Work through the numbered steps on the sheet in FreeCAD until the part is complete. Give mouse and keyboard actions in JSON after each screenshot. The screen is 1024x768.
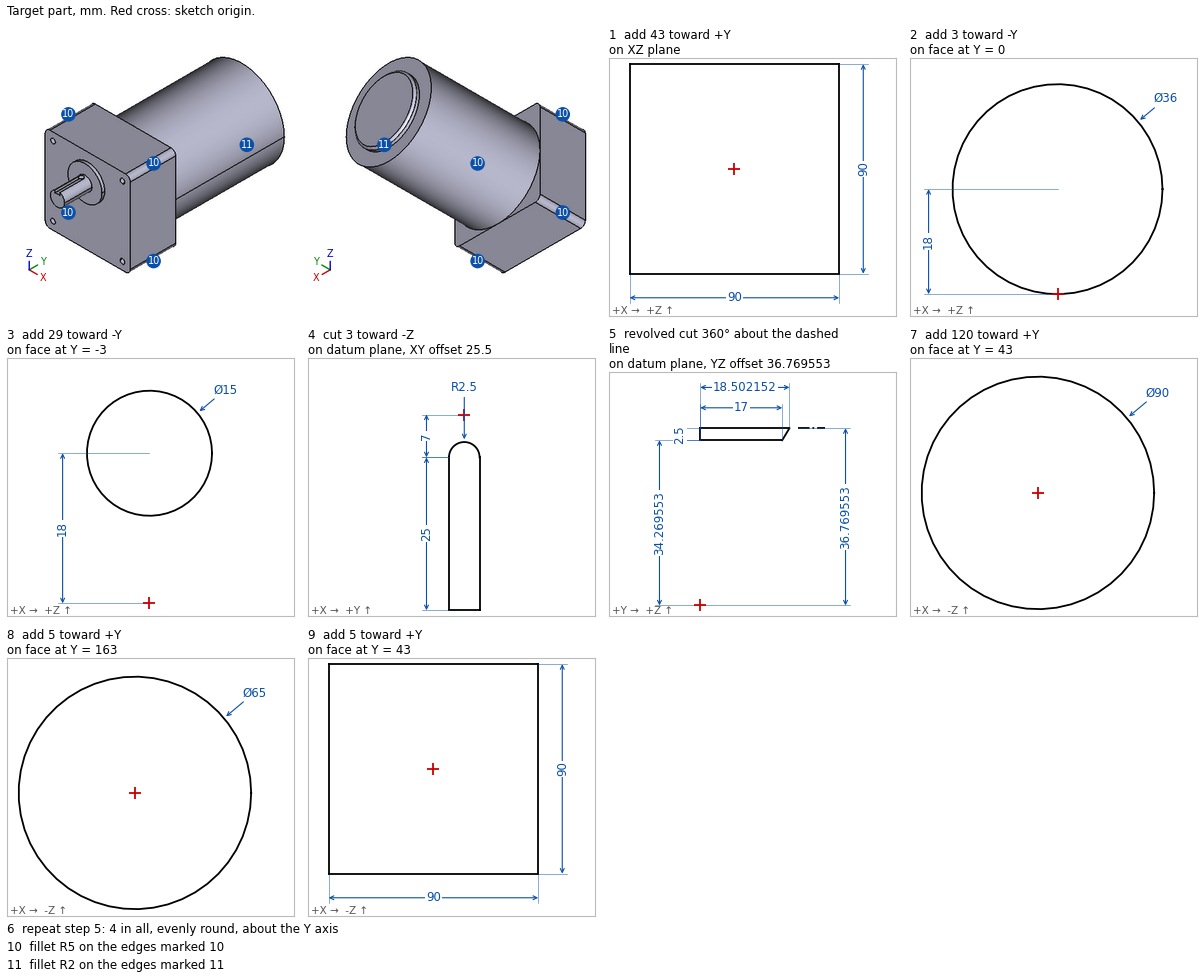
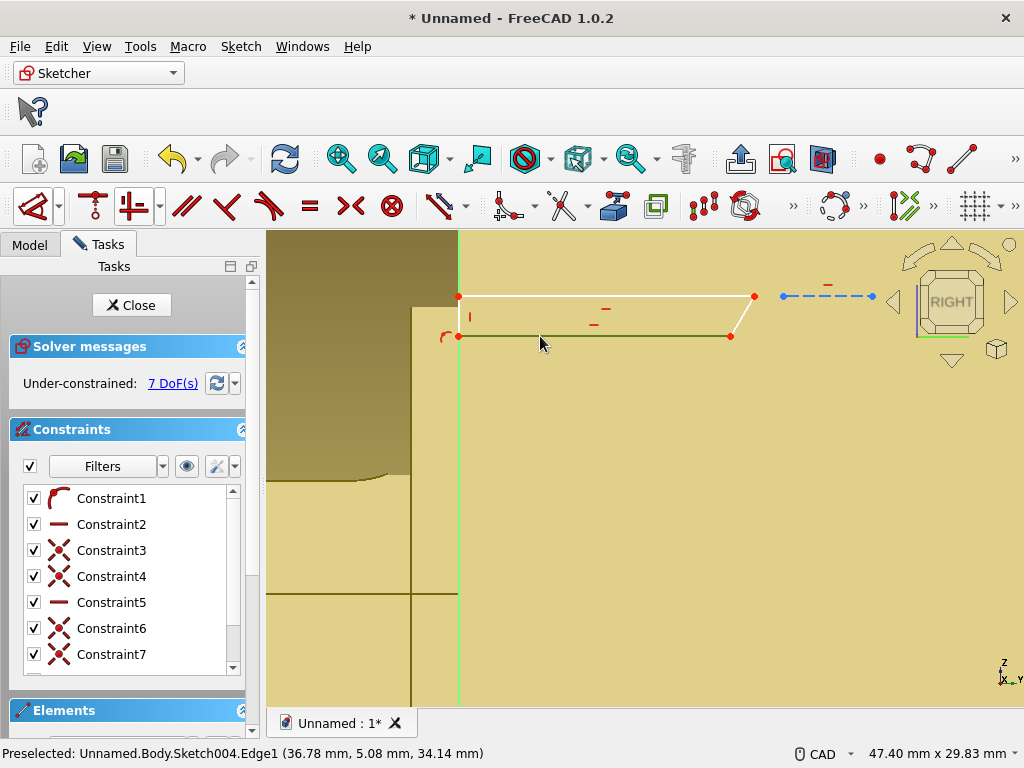
{"action": "left_click", "coordinate": [58, 206]}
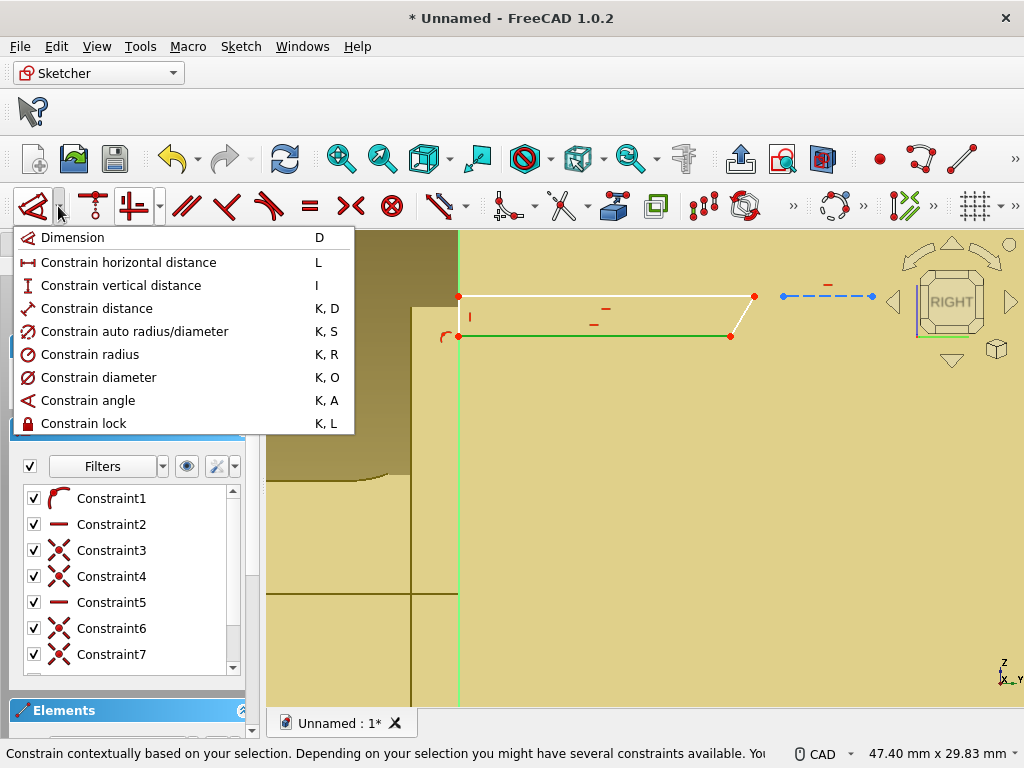
{"action": "left_click", "coordinate": [184, 262]}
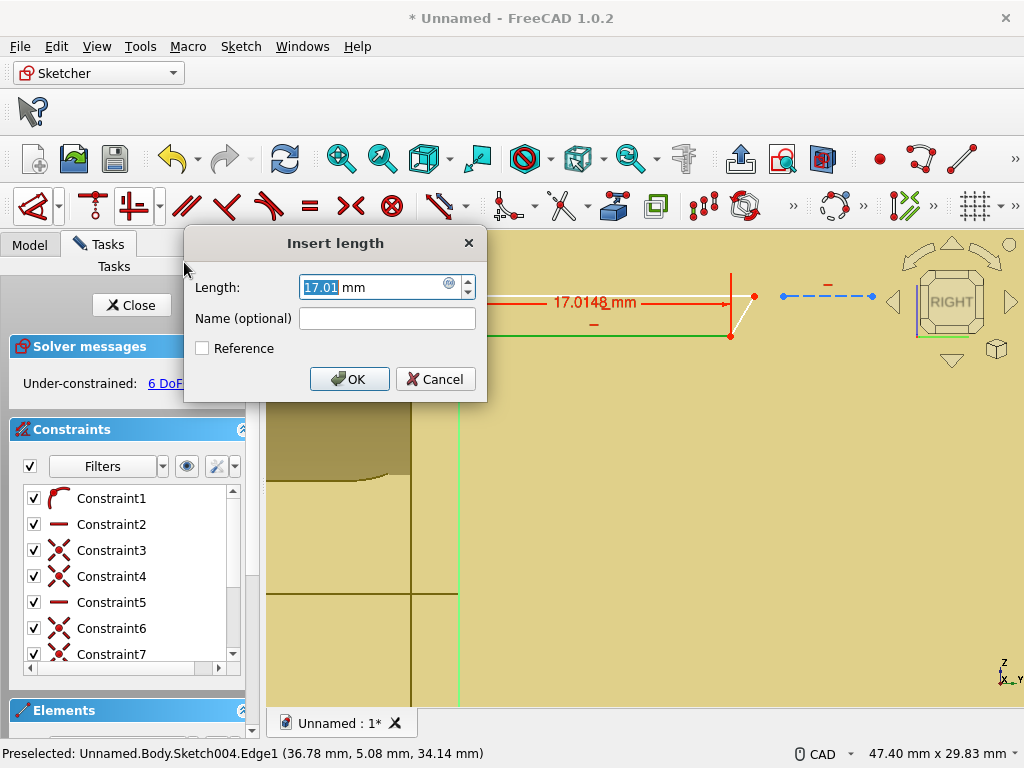
{"action": "type", "text": "17"}
{"action": "key", "text": "Return"}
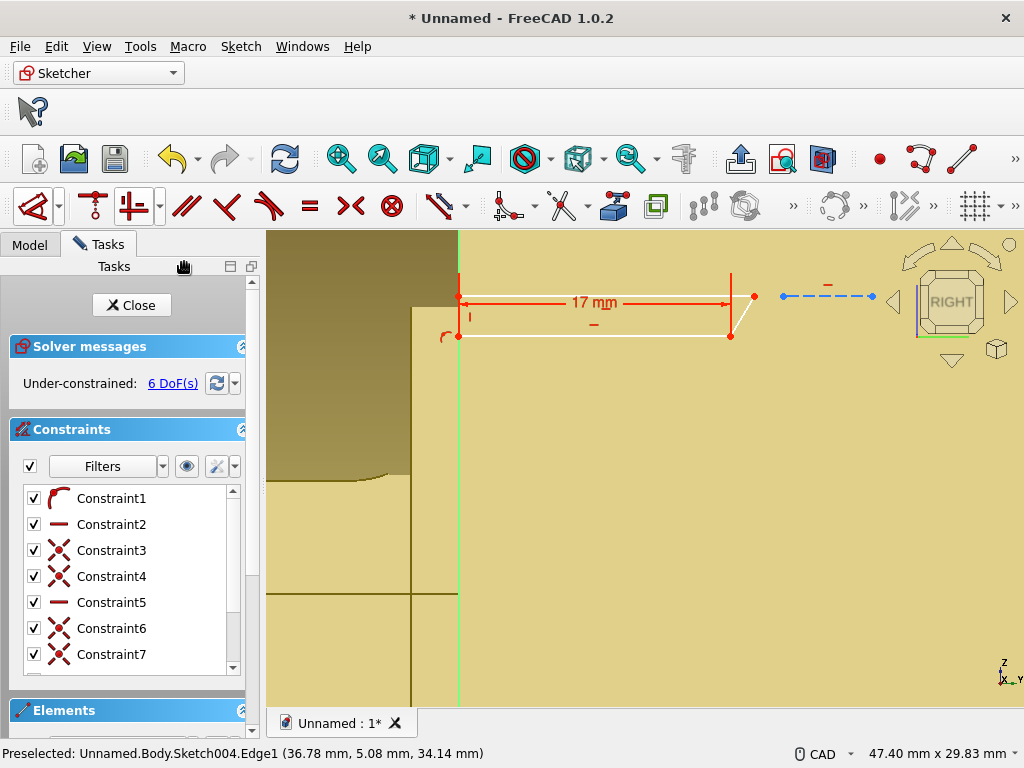
{"action": "left_click", "coordinate": [459, 308]}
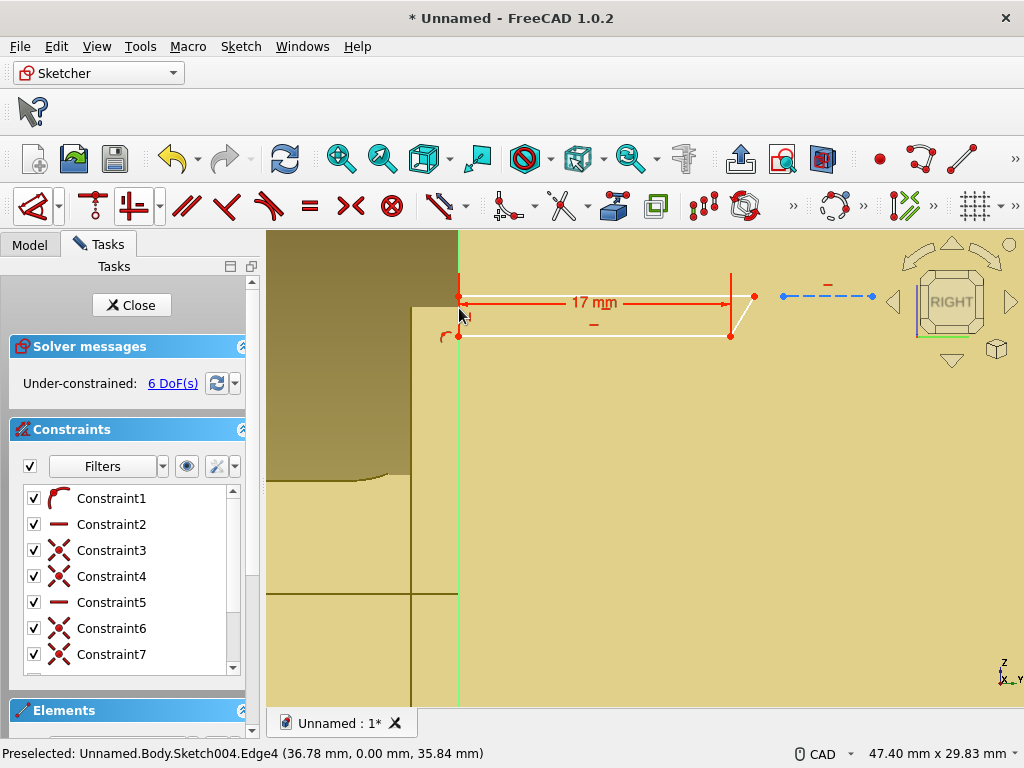
{"action": "key", "text": "i"}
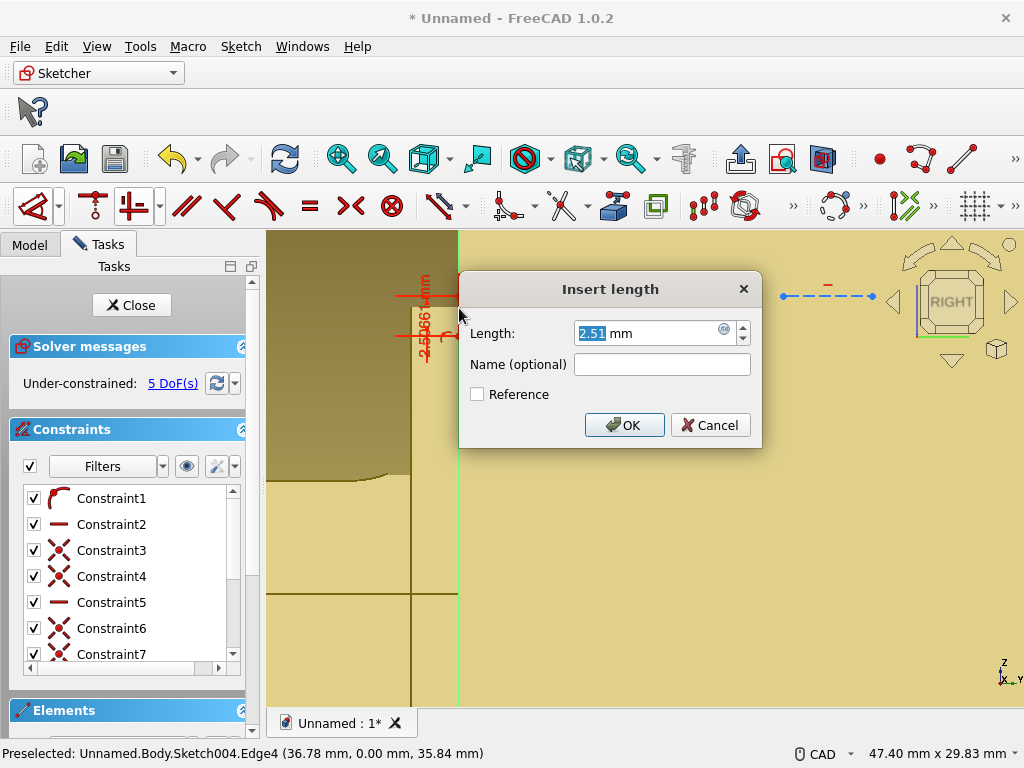
{"action": "type", "text": "2.5"}
{"action": "key", "text": "Return"}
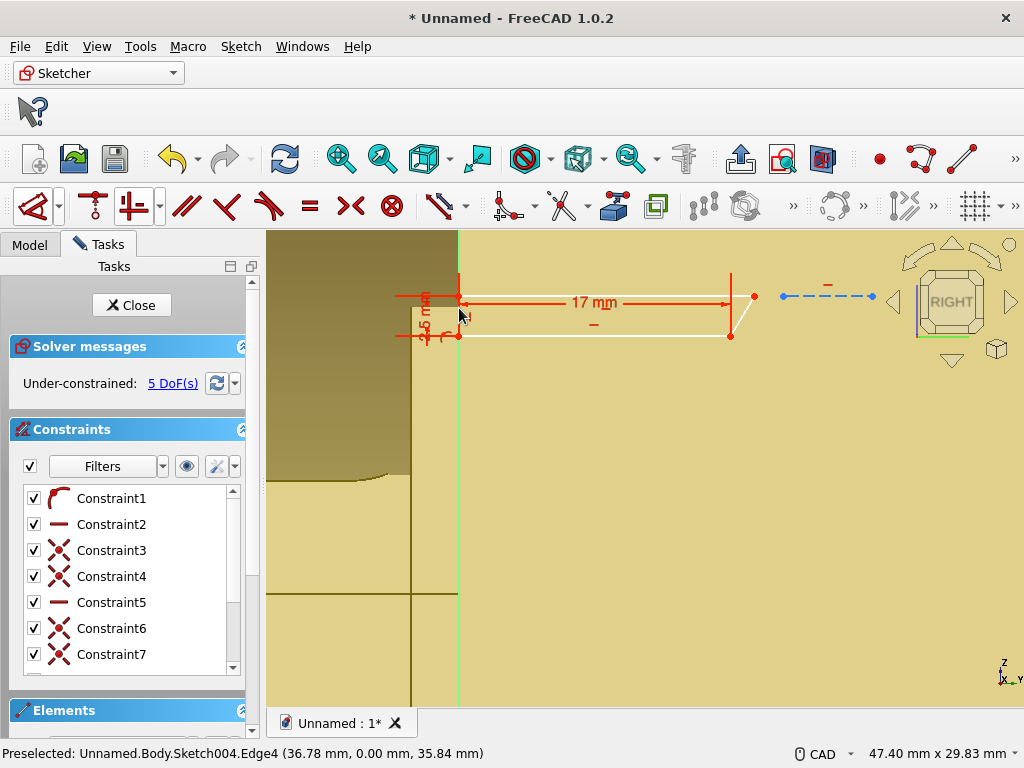
{"action": "left_click", "coordinate": [666, 296]}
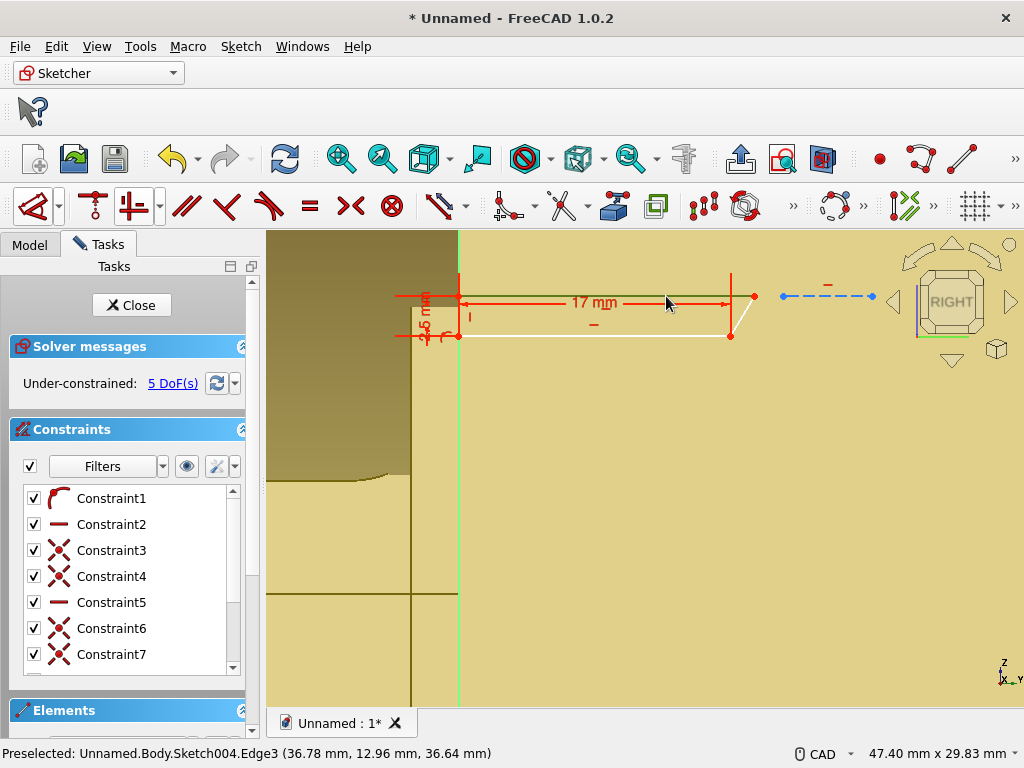
{"action": "left_click", "coordinate": [58, 206]}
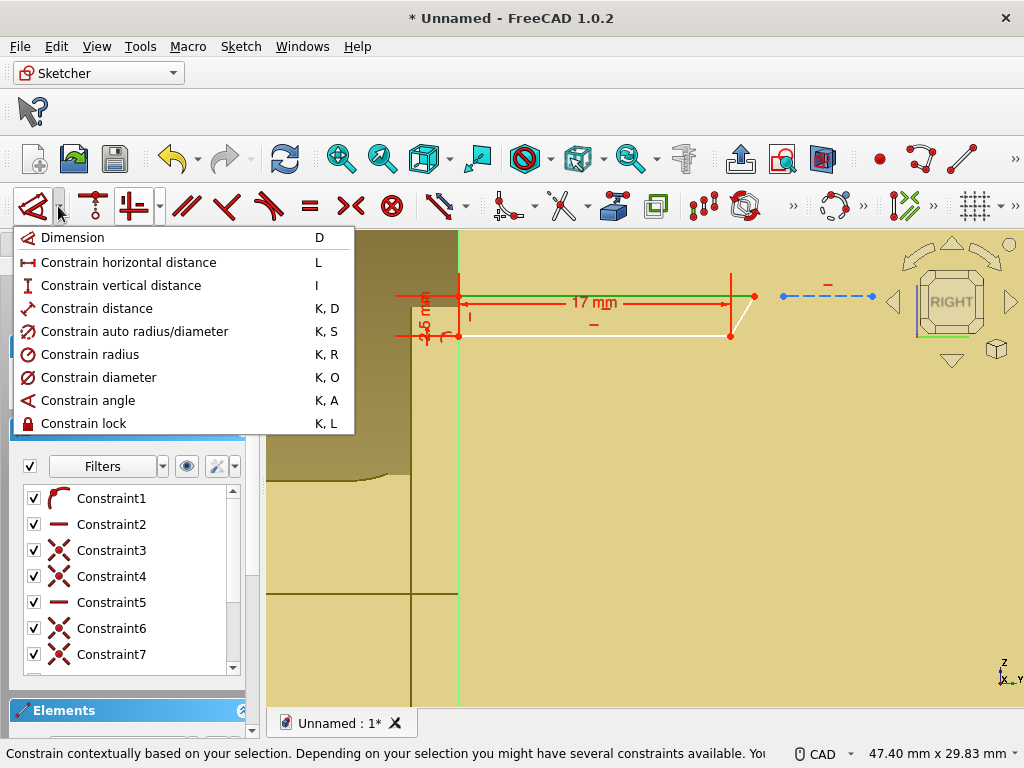
{"action": "left_click", "coordinate": [184, 262]}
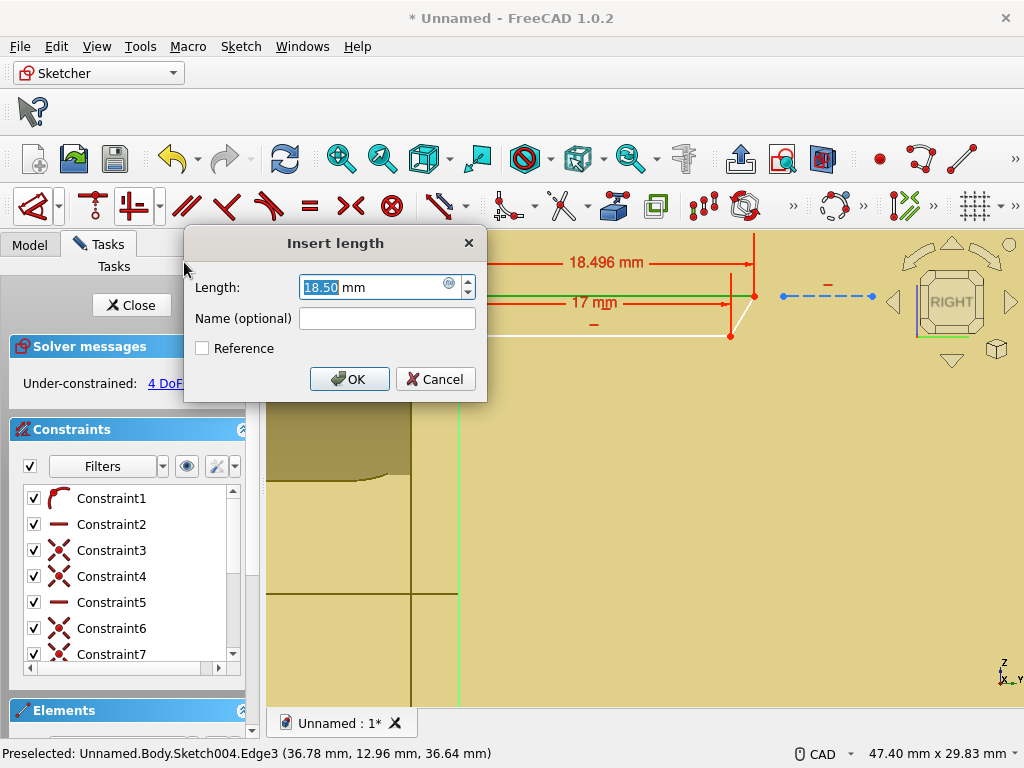
{"action": "type", "text": "18.502152"}
{"action": "key", "text": "Return"}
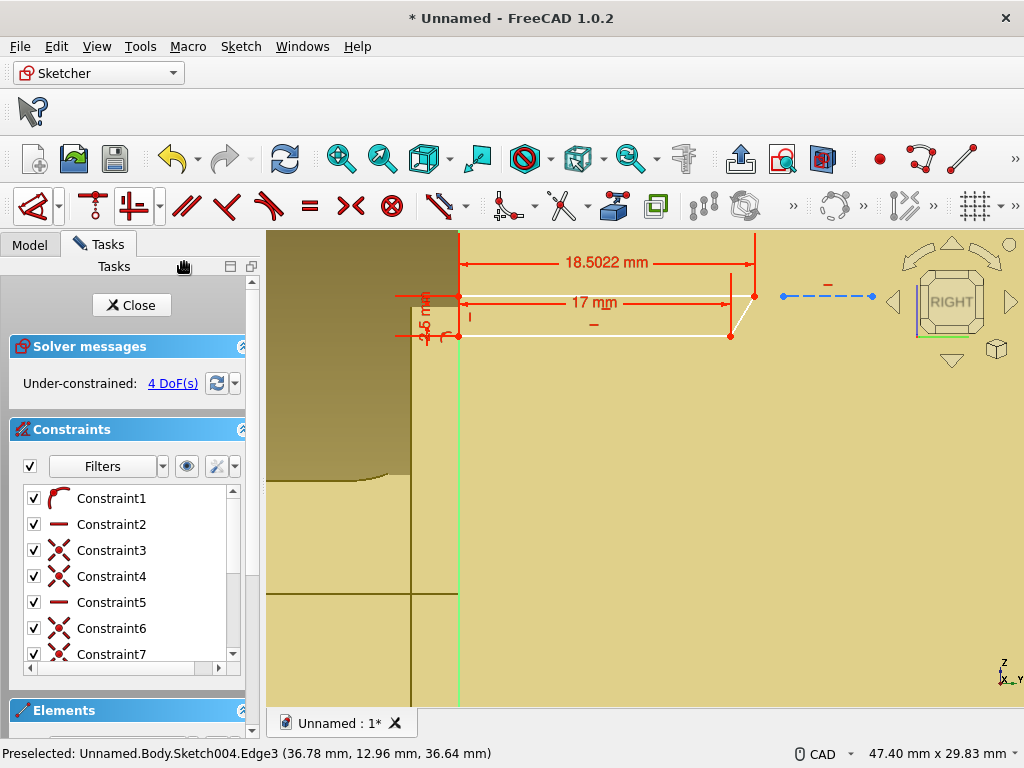
{"action": "left_click", "coordinate": [459, 336]}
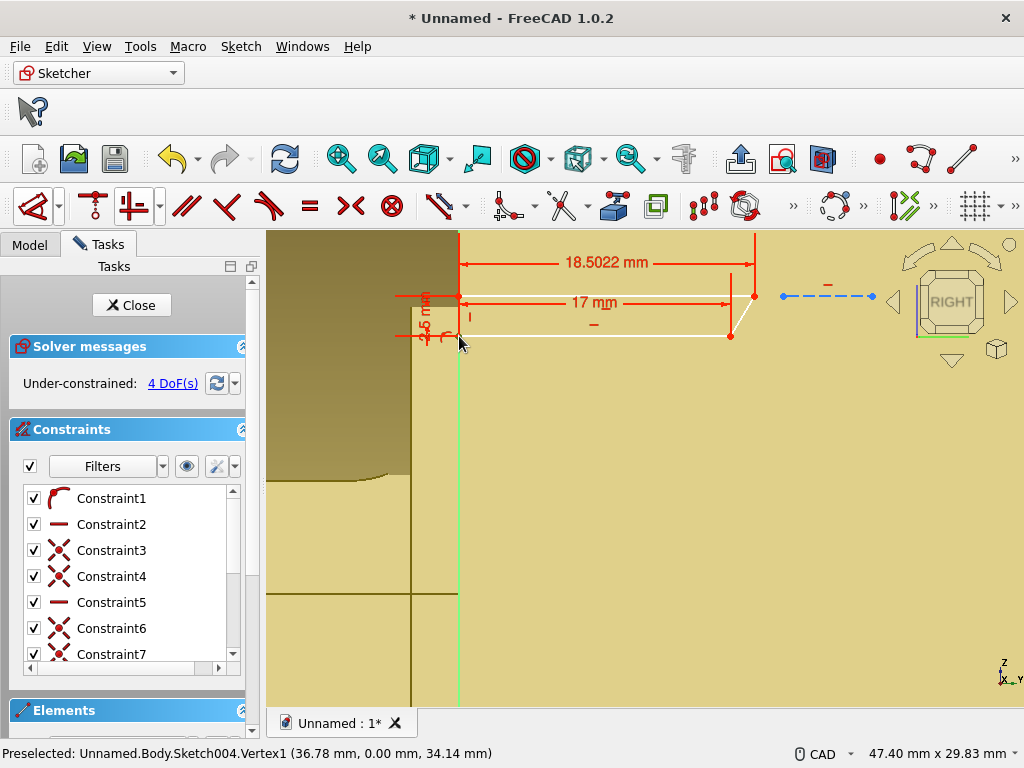
{"action": "key", "text": "i"}